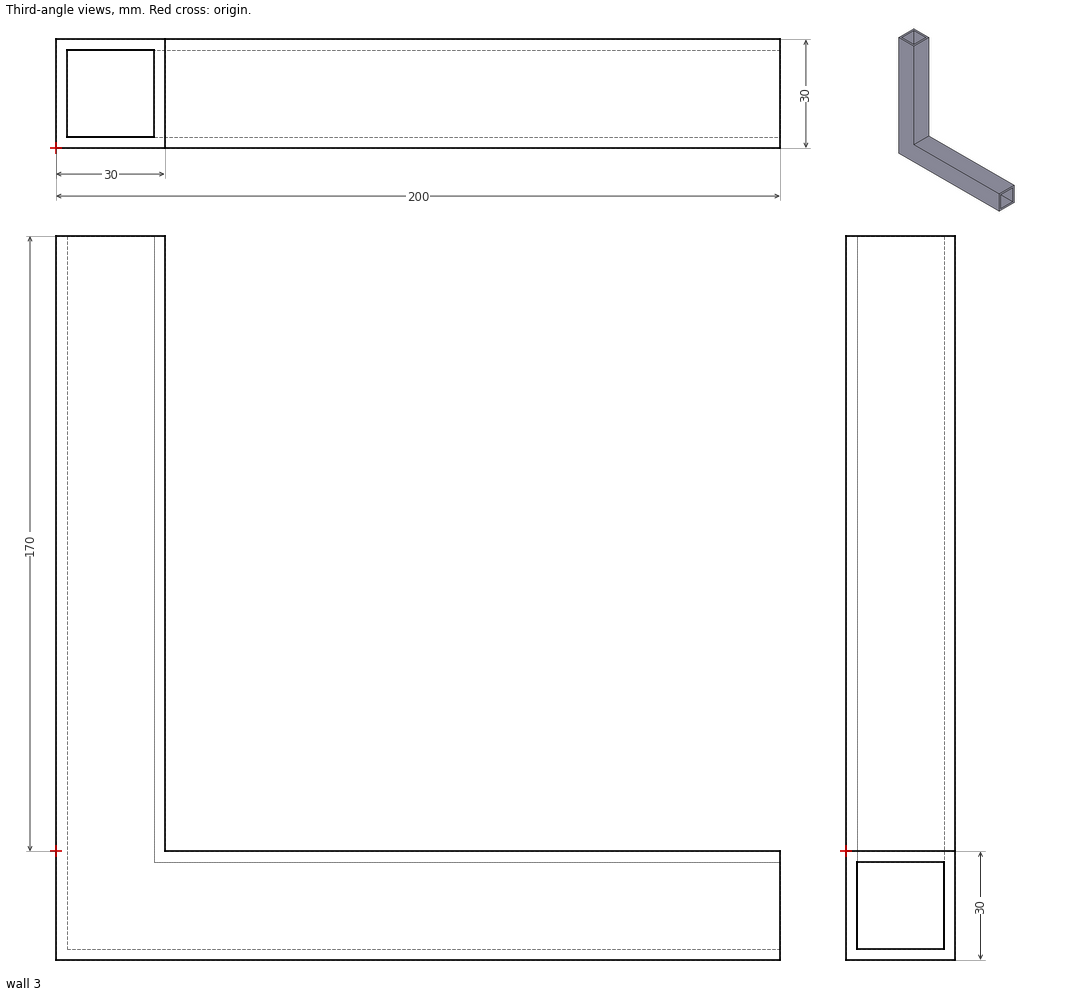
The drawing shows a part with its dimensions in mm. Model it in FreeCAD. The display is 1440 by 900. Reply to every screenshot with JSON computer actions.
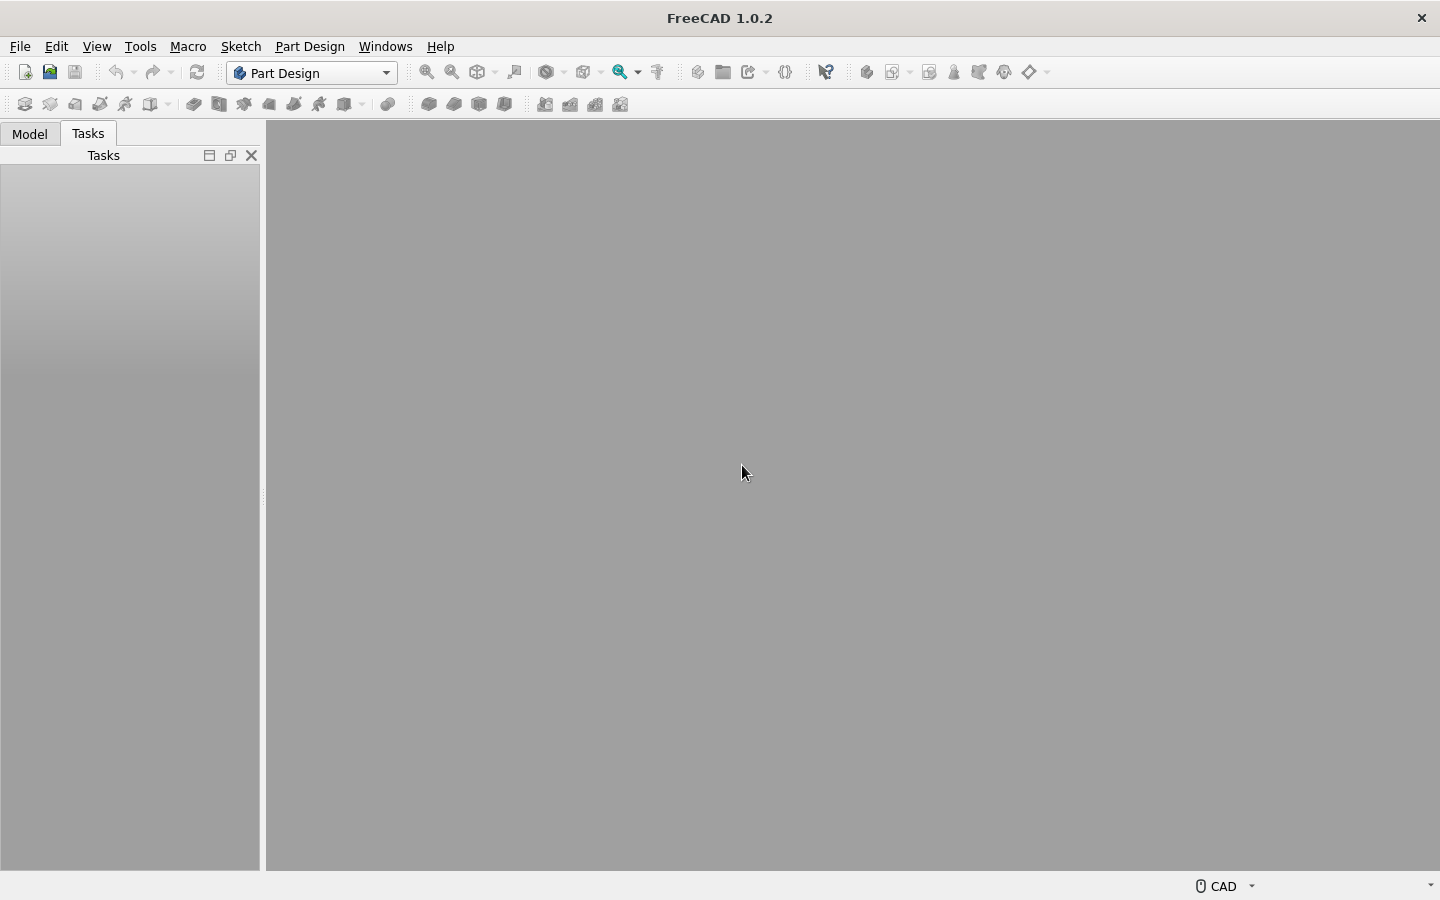
{"action": "key", "text": "ctrl+n"}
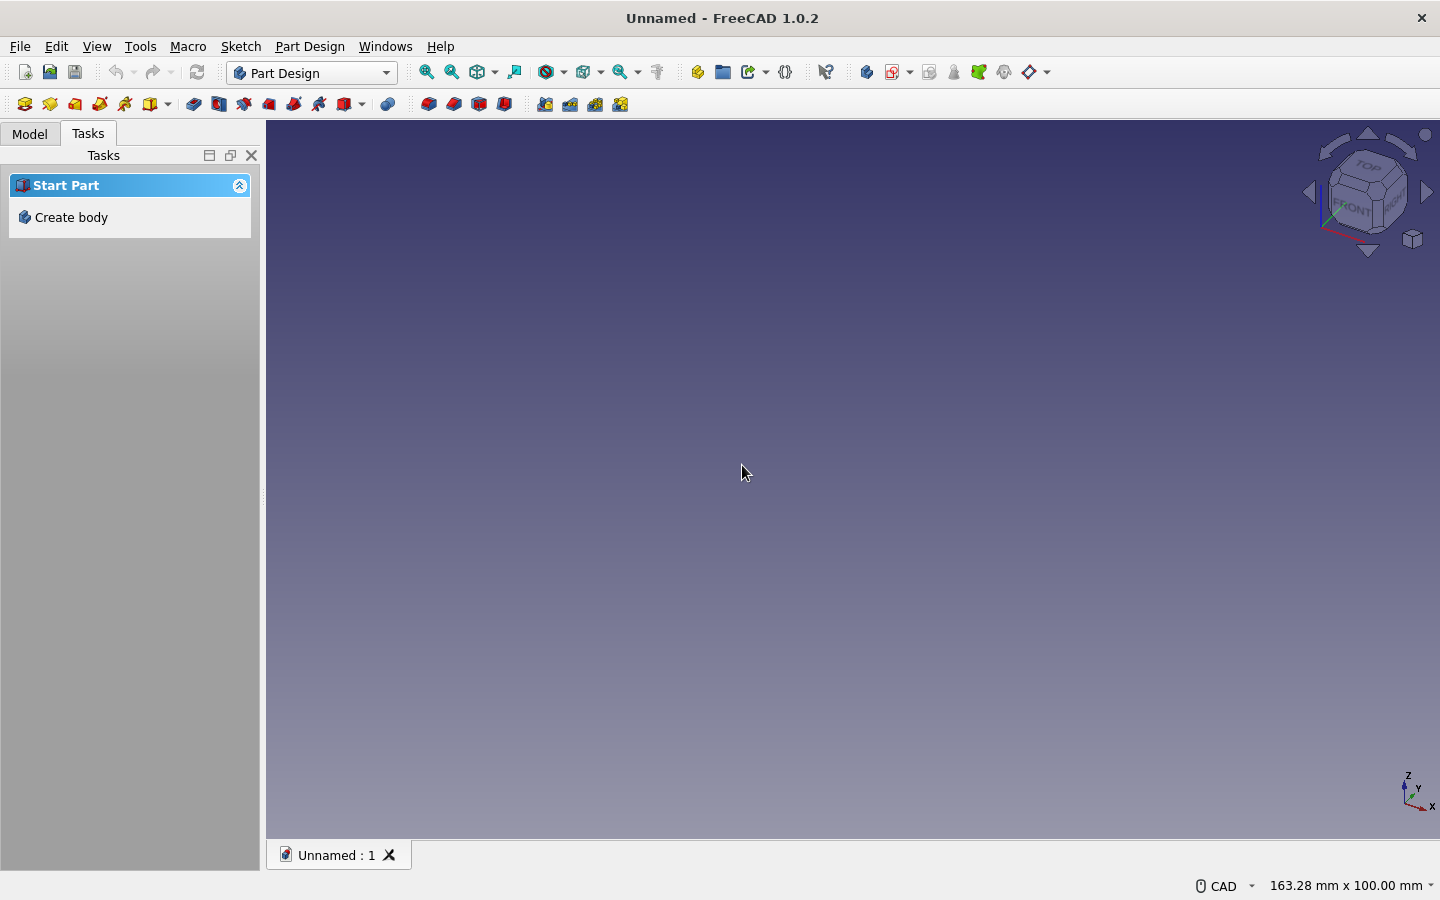
{"action": "left_click", "coordinate": [892, 72]}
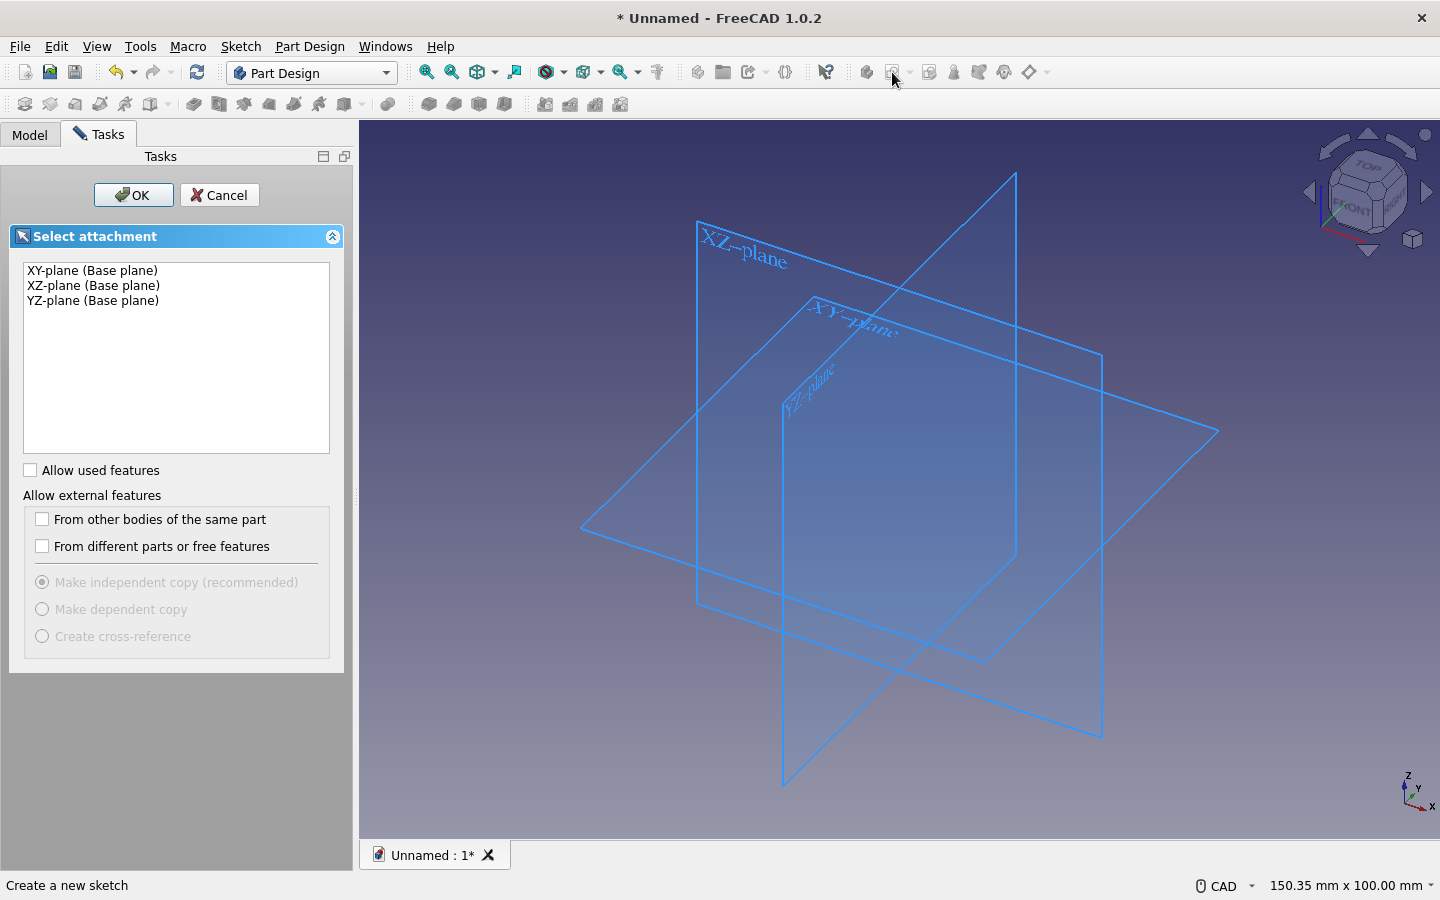
{"action": "left_click", "coordinate": [84, 270]}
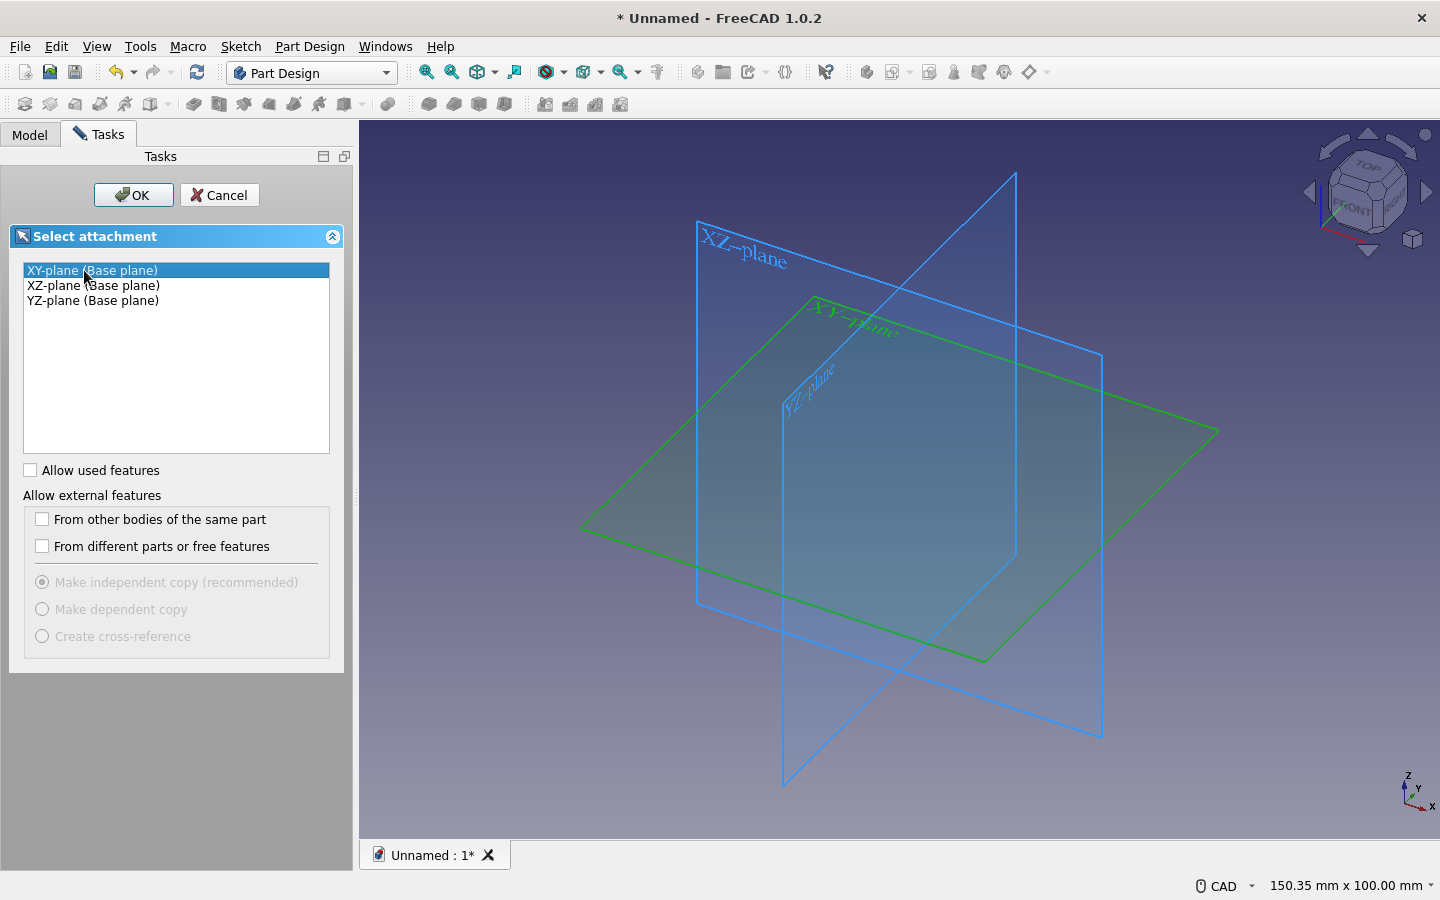
{"action": "left_click", "coordinate": [134, 195]}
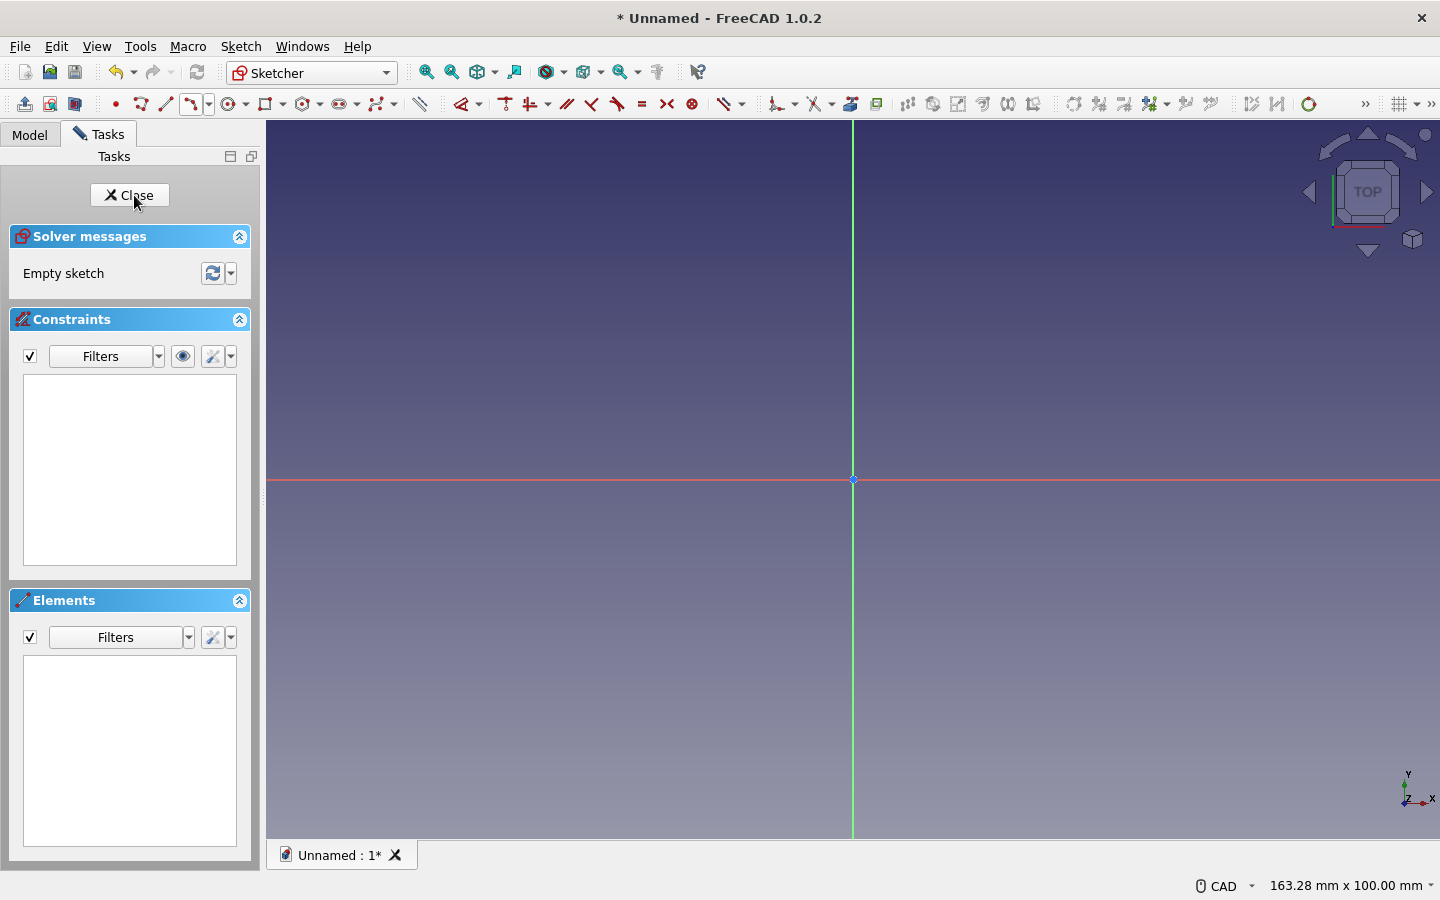
{"action": "scroll", "coordinate": [294, 568], "scroll_direction": "down", "scroll_amount": 4}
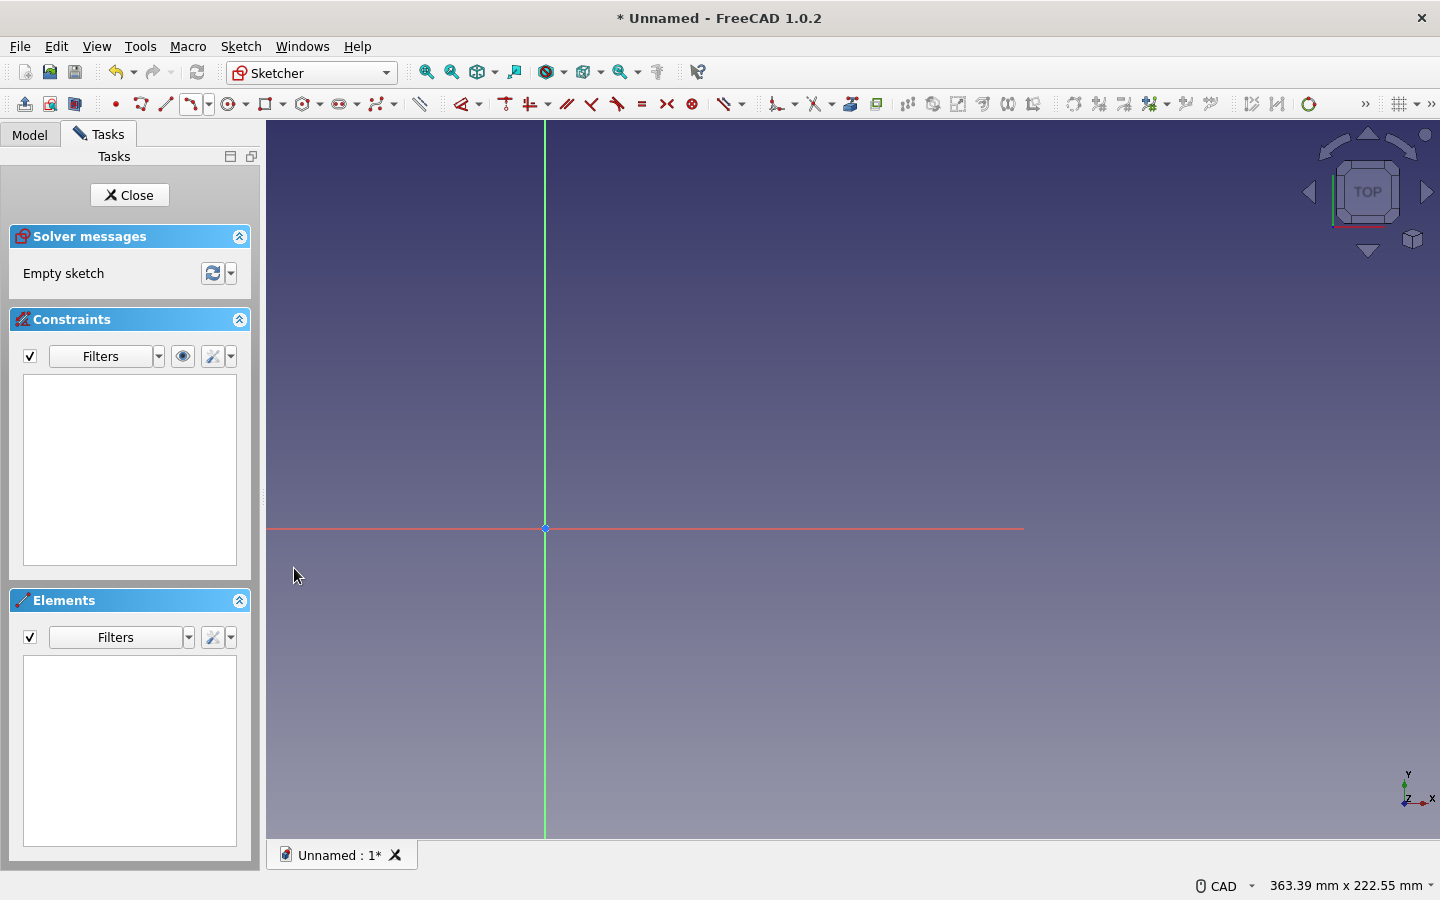
{"action": "left_click", "coordinate": [264, 104]}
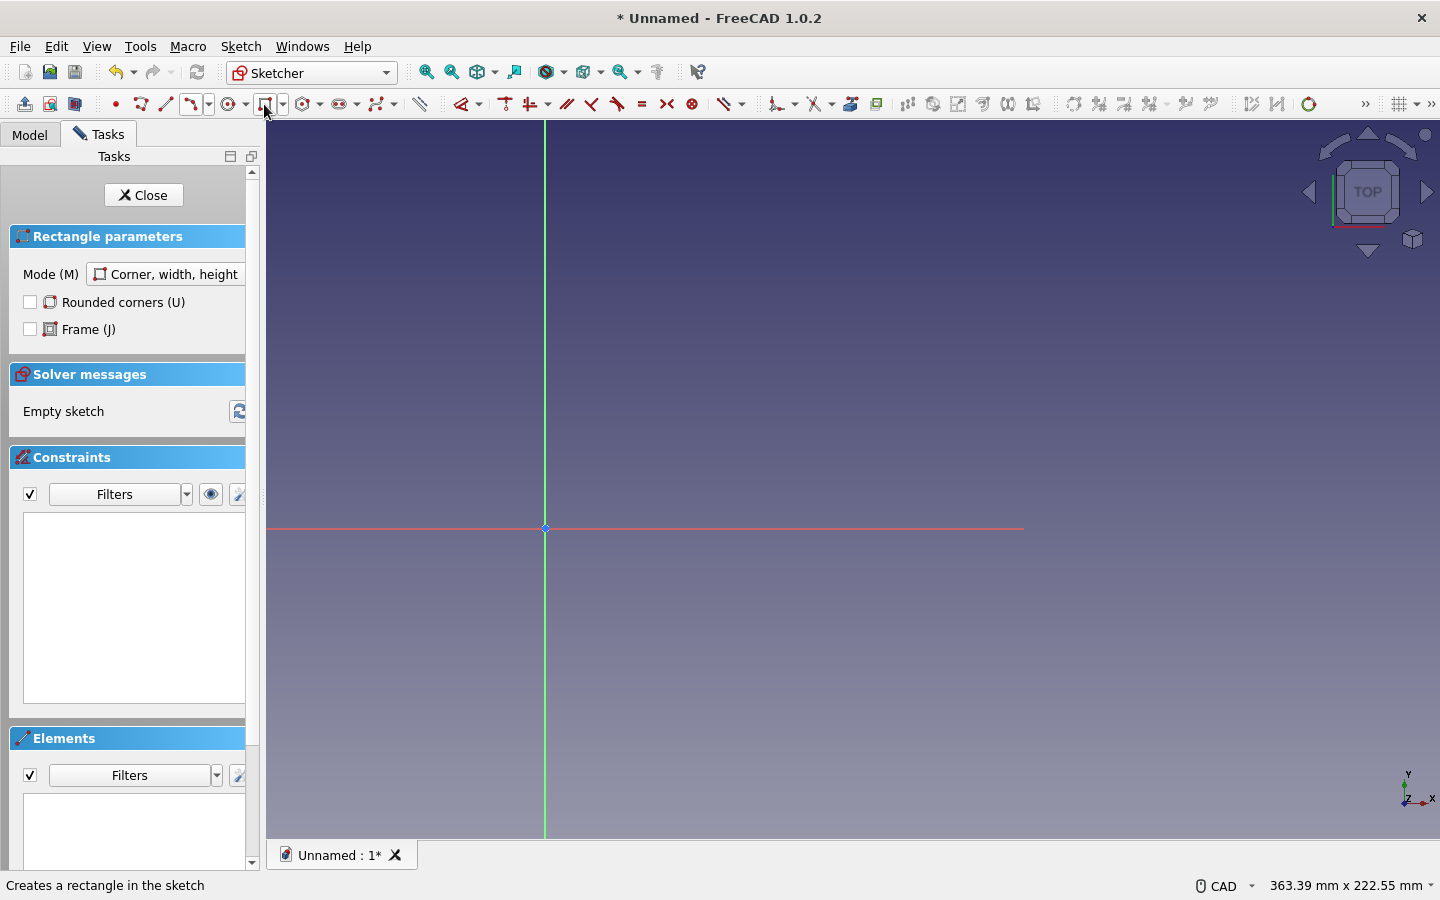
{"action": "left_click", "coordinate": [545, 529]}
{"action": "mouse_move", "coordinate": [1191, 432]}